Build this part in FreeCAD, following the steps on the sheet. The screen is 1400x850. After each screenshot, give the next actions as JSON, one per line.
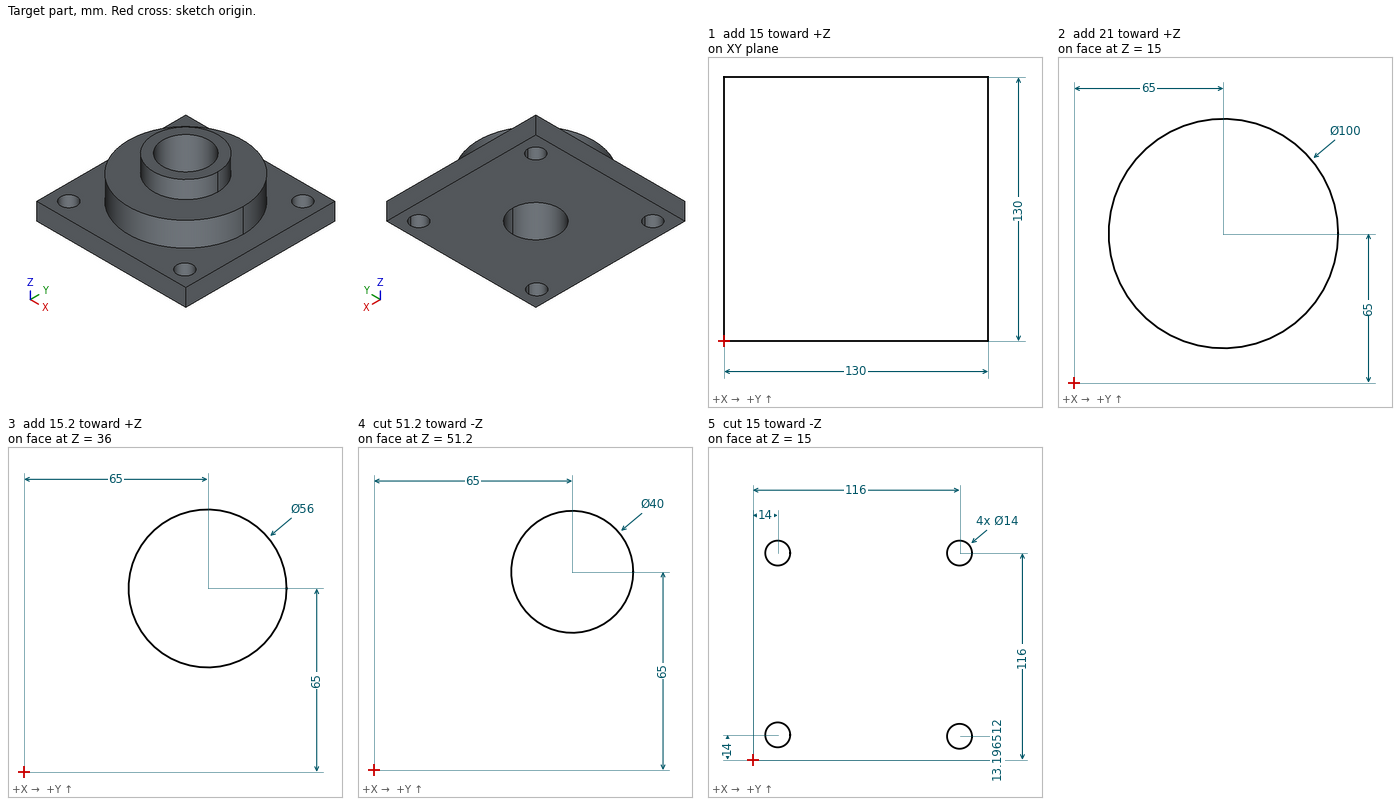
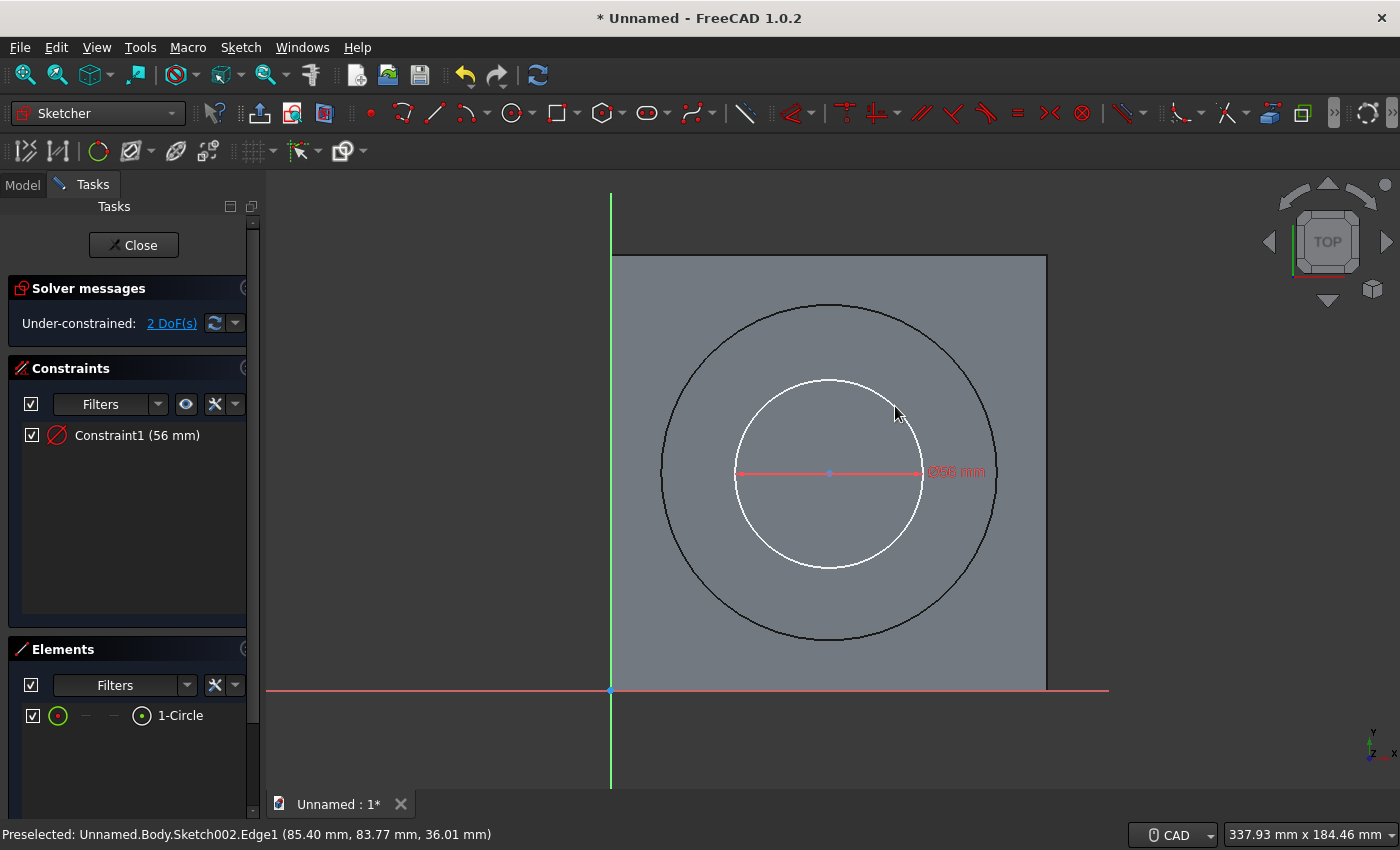
{"action": "key", "text": "d"}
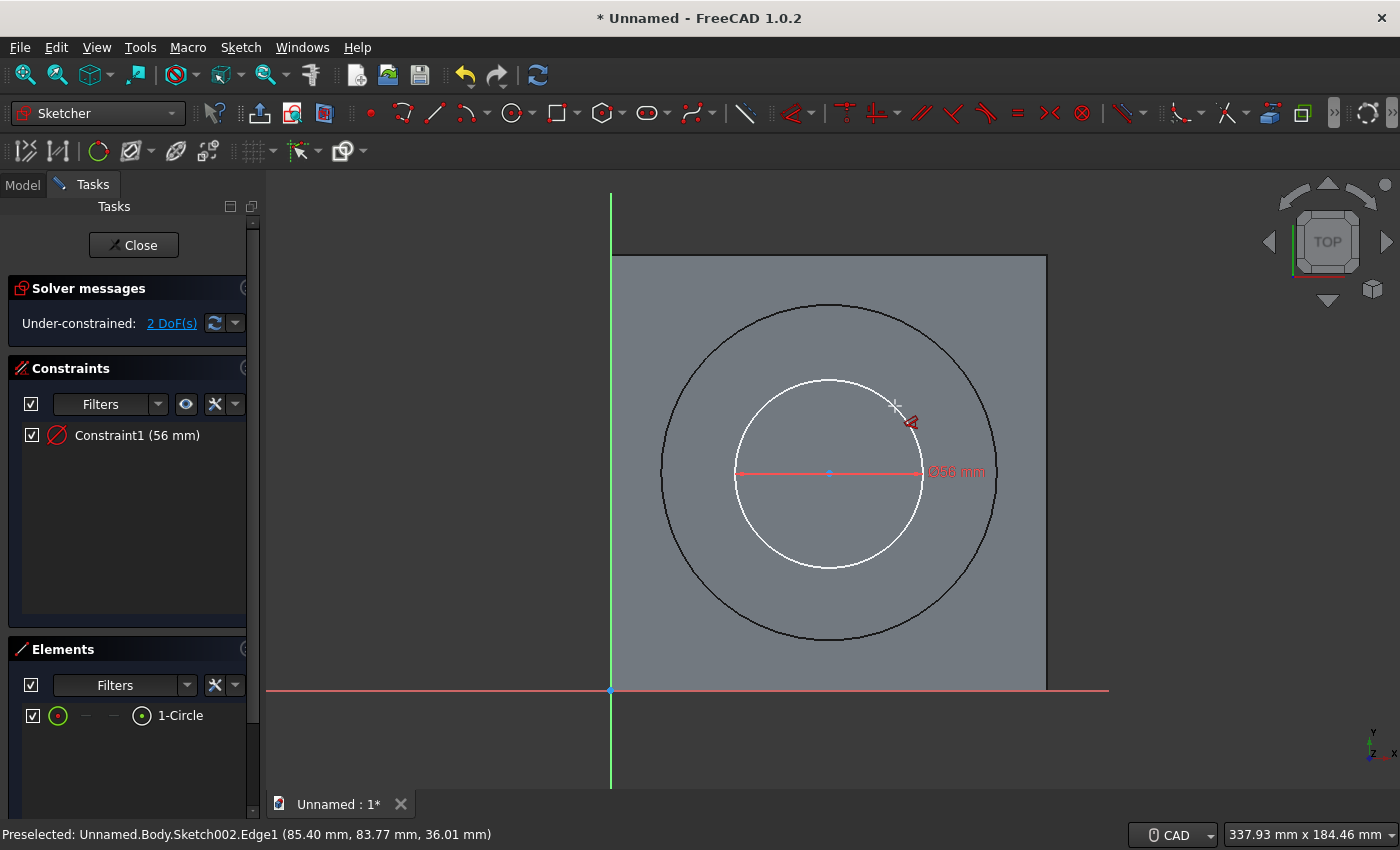
{"action": "left_click", "coordinate": [829, 474]}
{"action": "left_click", "coordinate": [720, 725]}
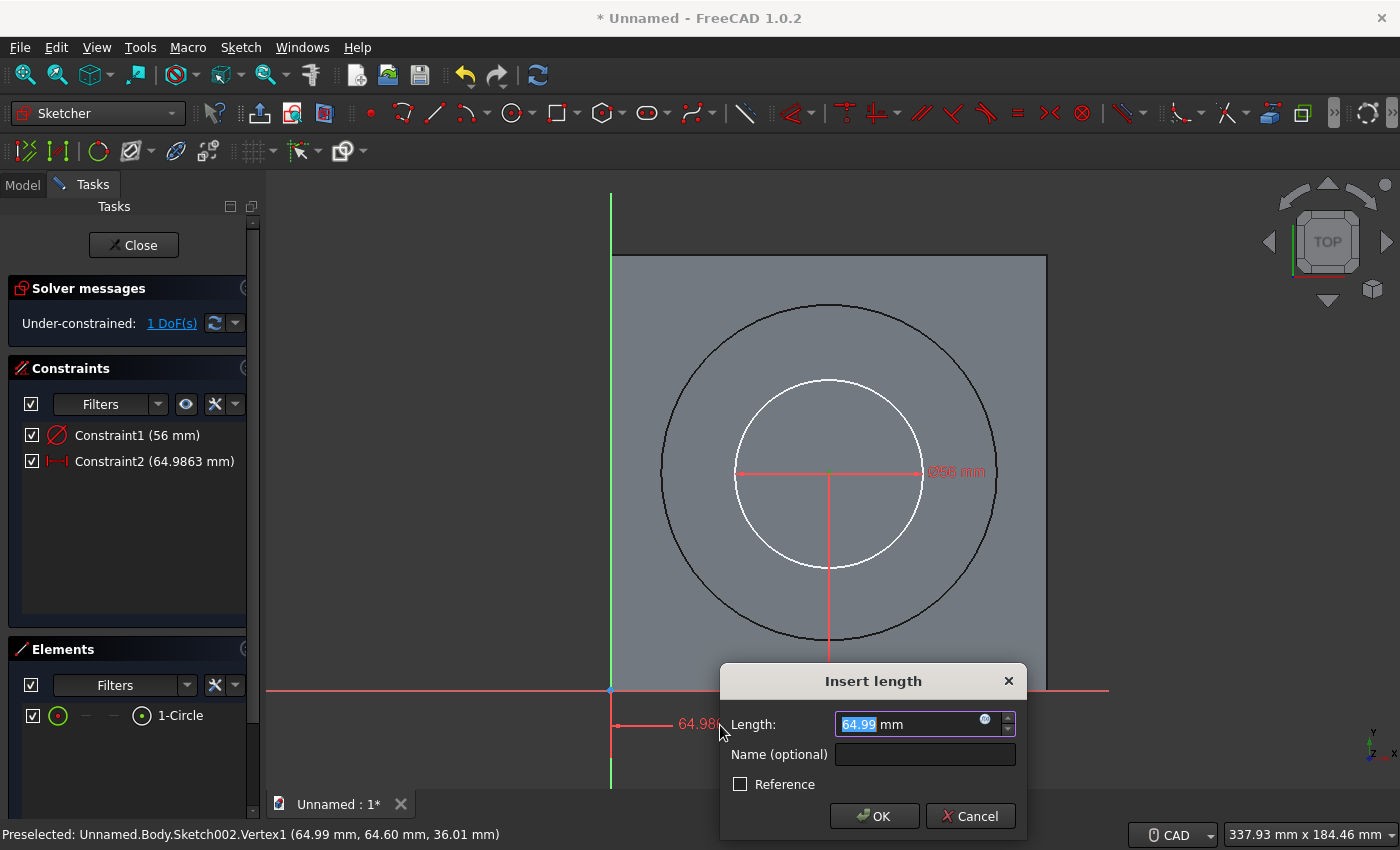
{"action": "type", "text": "65"}
{"action": "key", "text": "Return"}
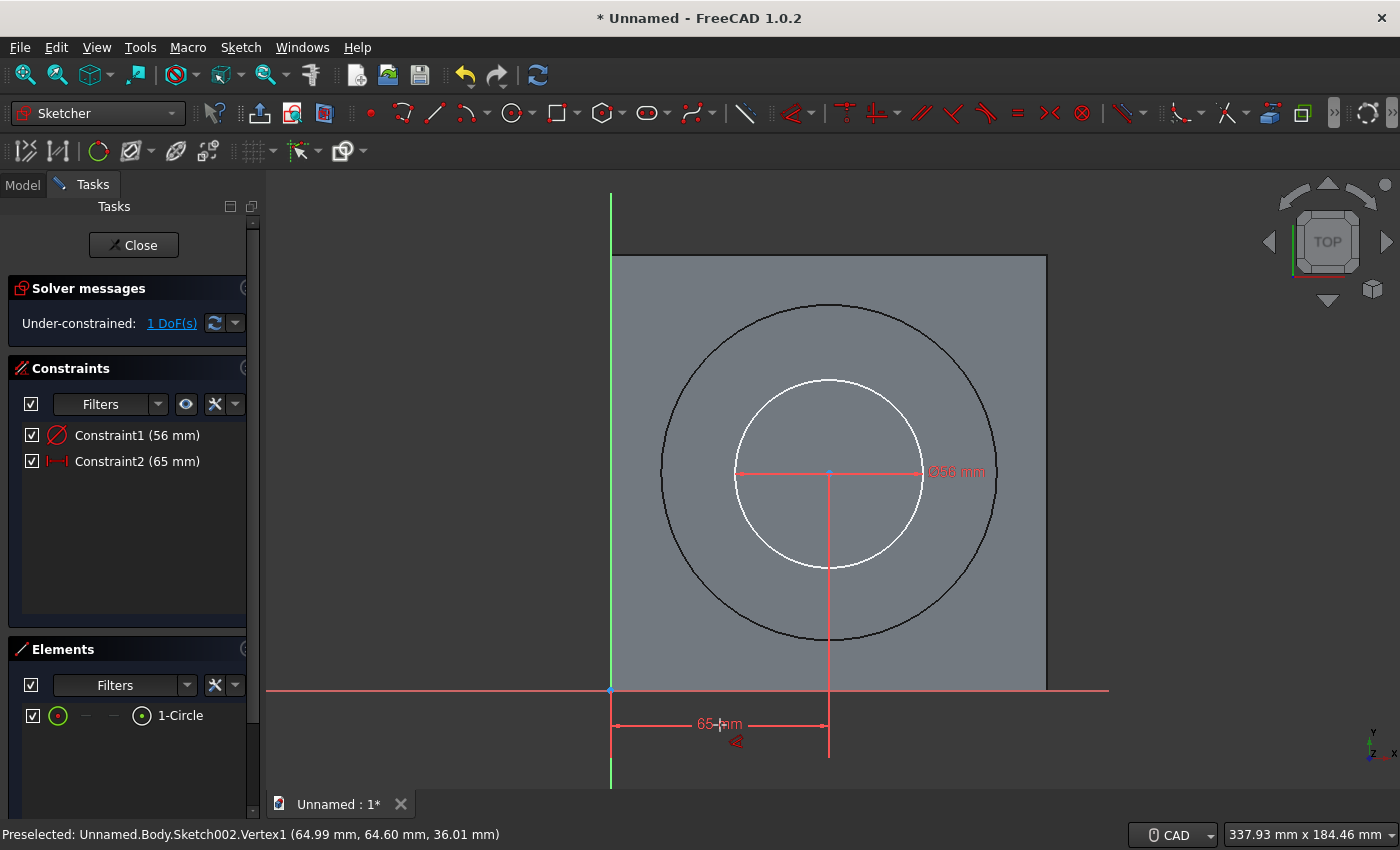
{"action": "left_click", "coordinate": [829, 474]}
{"action": "left_click", "coordinate": [577, 582]}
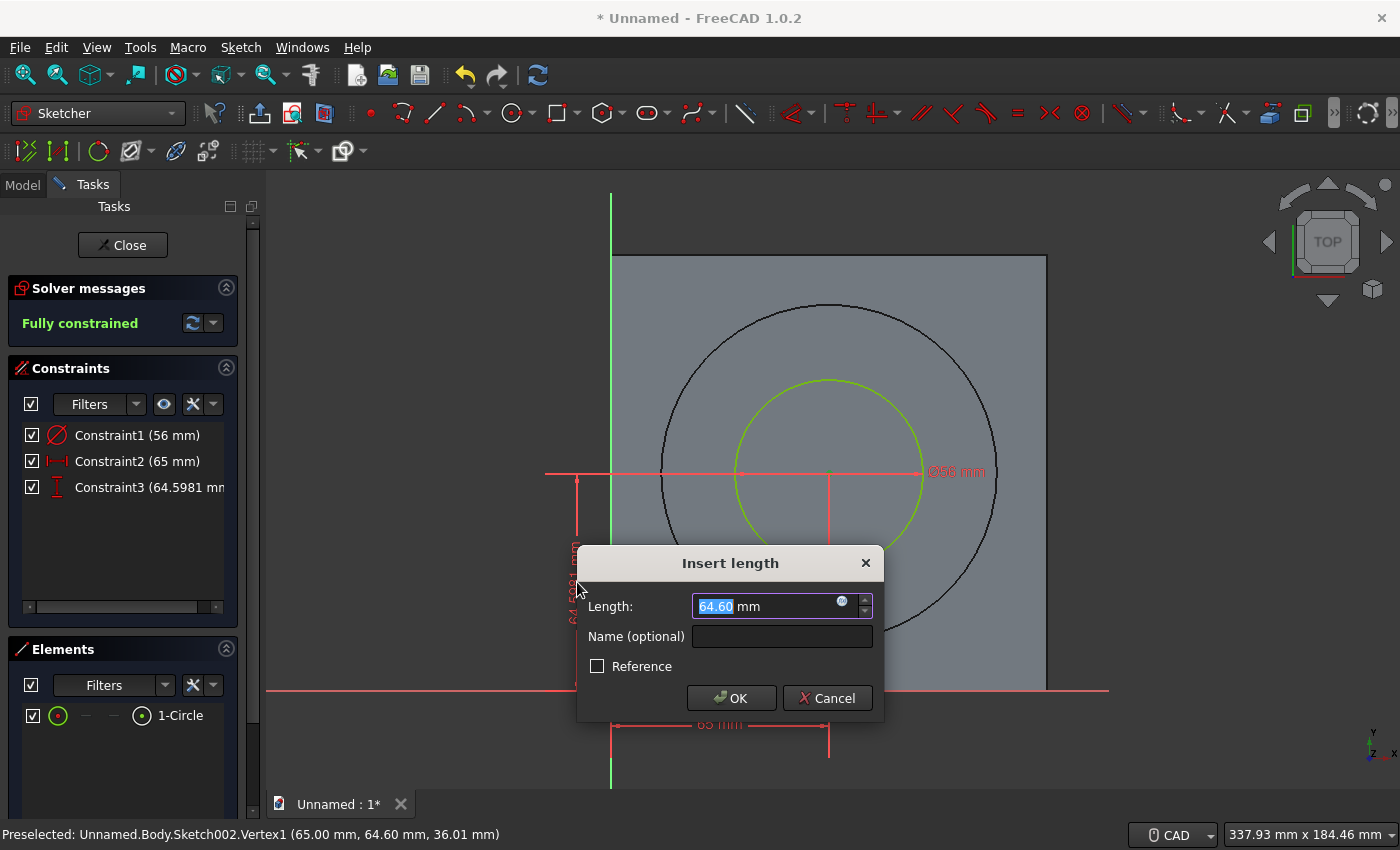
{"action": "type", "text": "65"}
{"action": "key", "text": "Return"}
{"action": "key", "text": "Escape"}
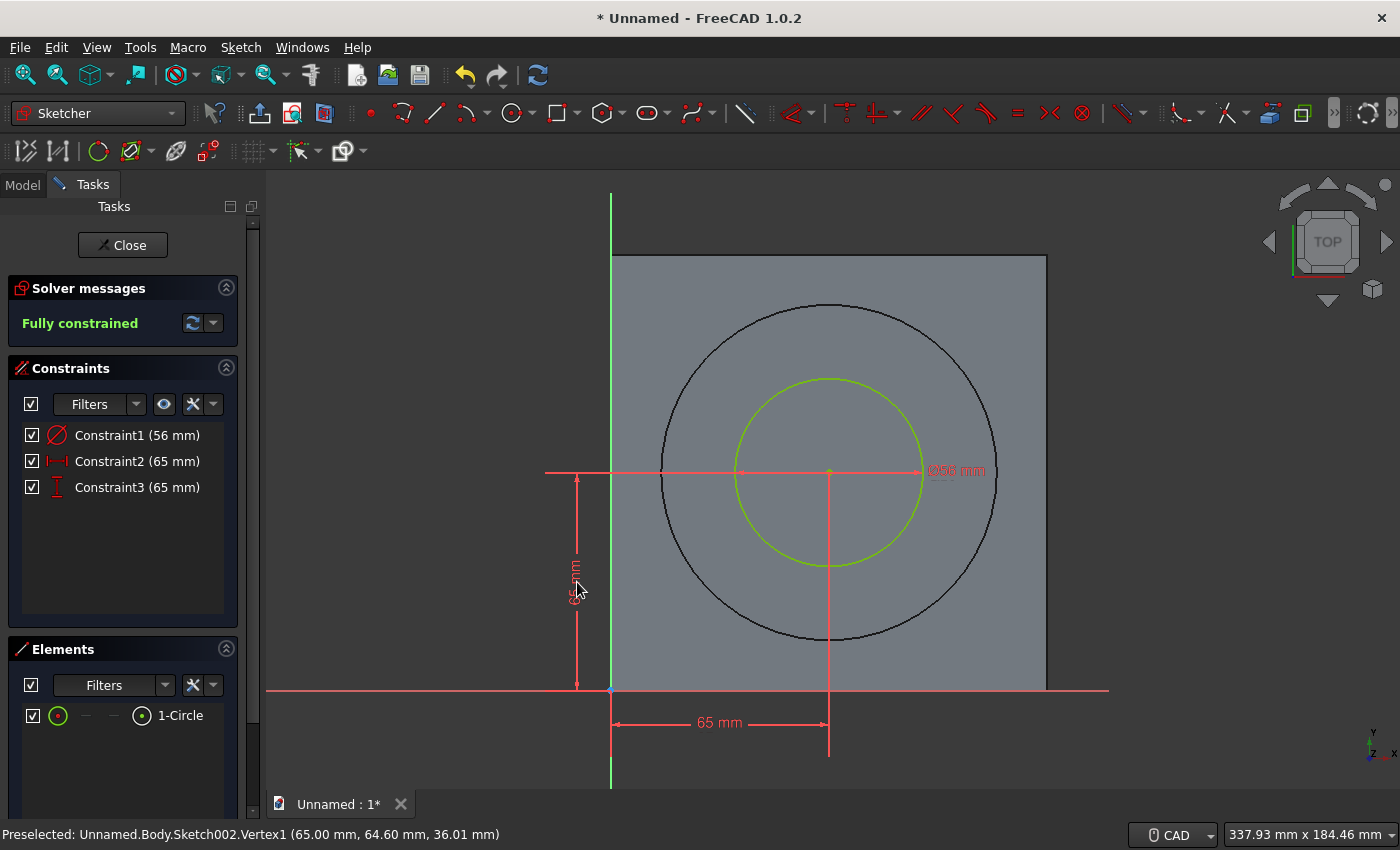
{"action": "left_click", "coordinate": [123, 245]}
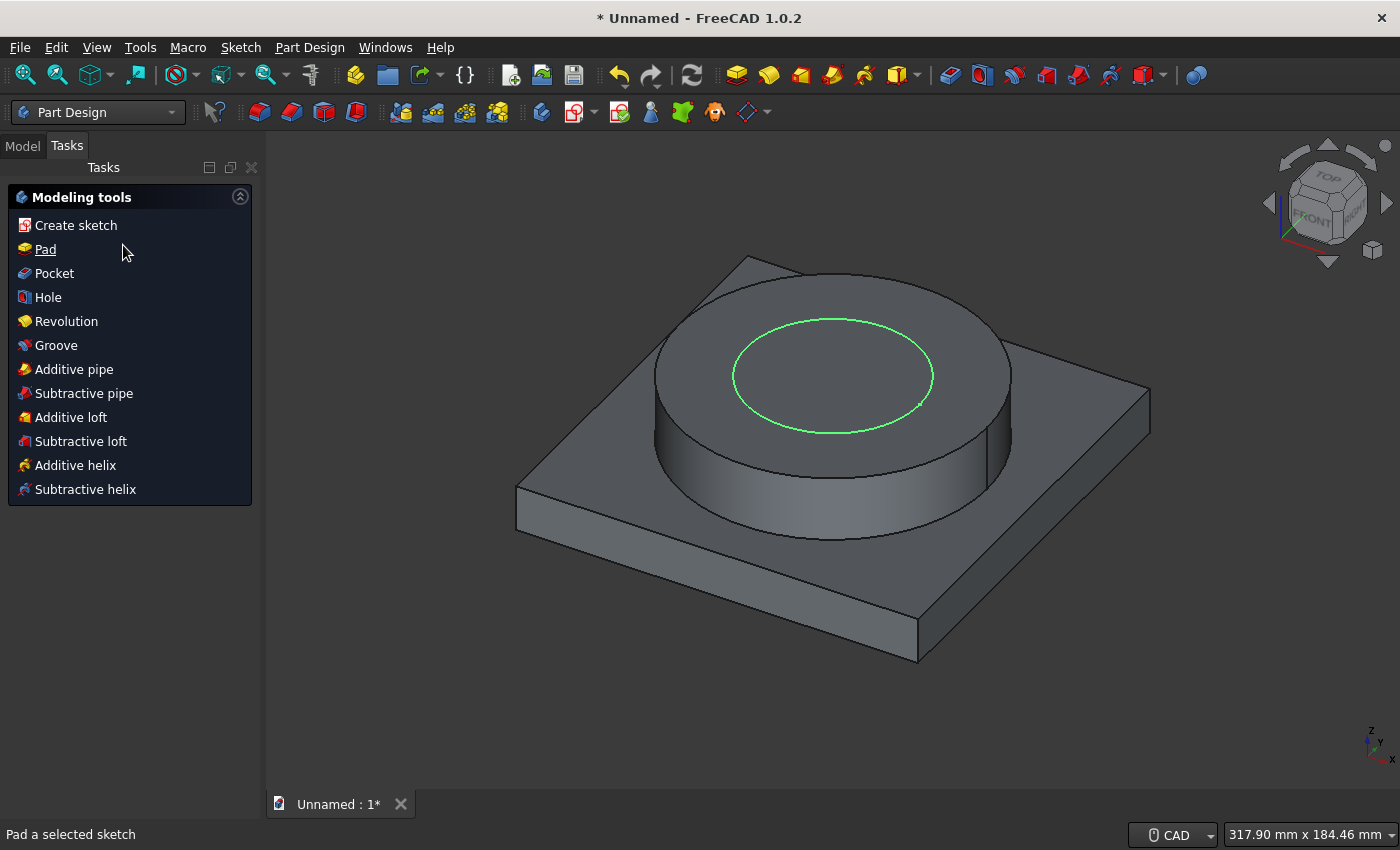
{"action": "left_click", "coordinate": [738, 76]}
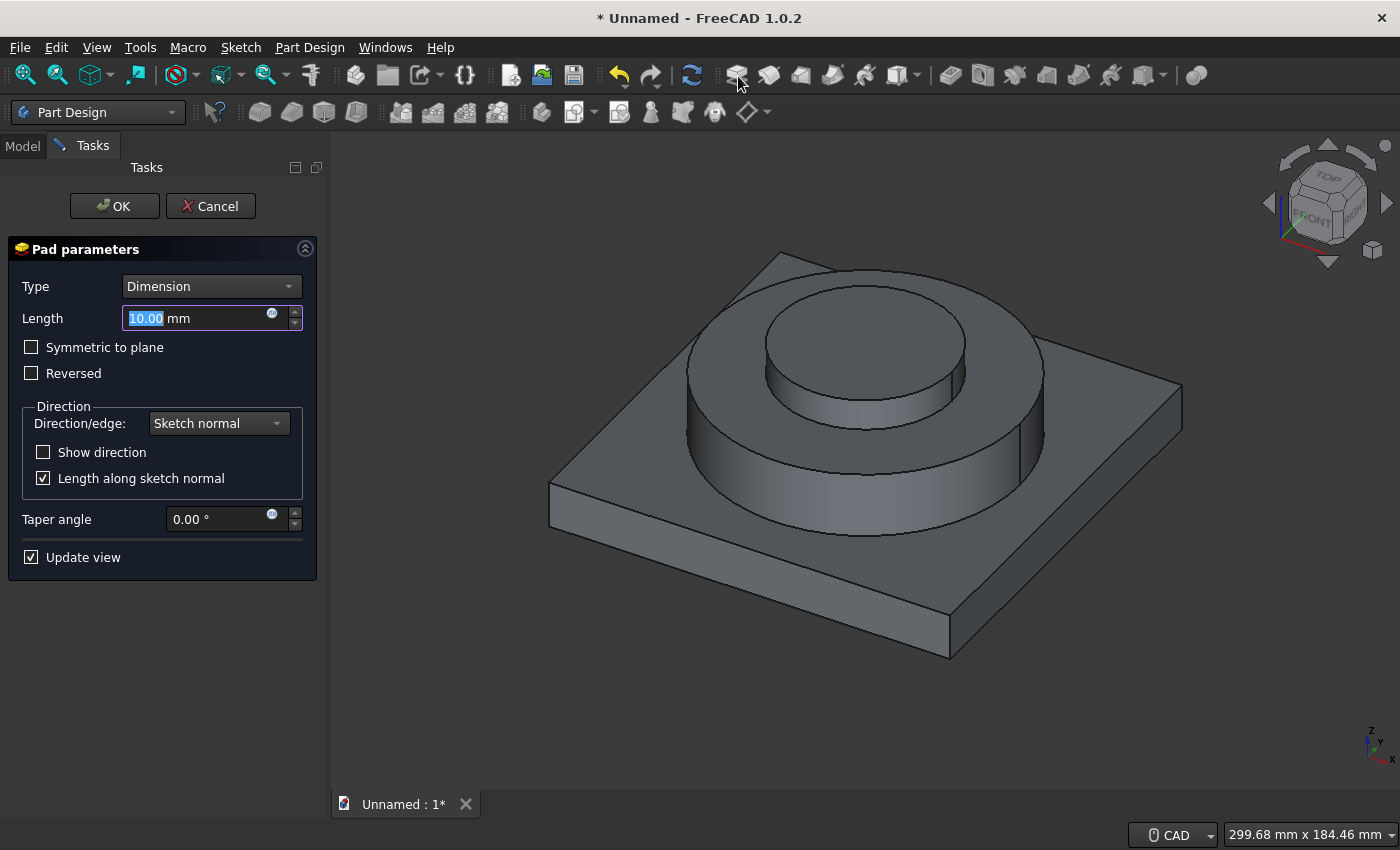
{"action": "type", "text": "15.2"}
{"action": "key", "text": "Tab"}